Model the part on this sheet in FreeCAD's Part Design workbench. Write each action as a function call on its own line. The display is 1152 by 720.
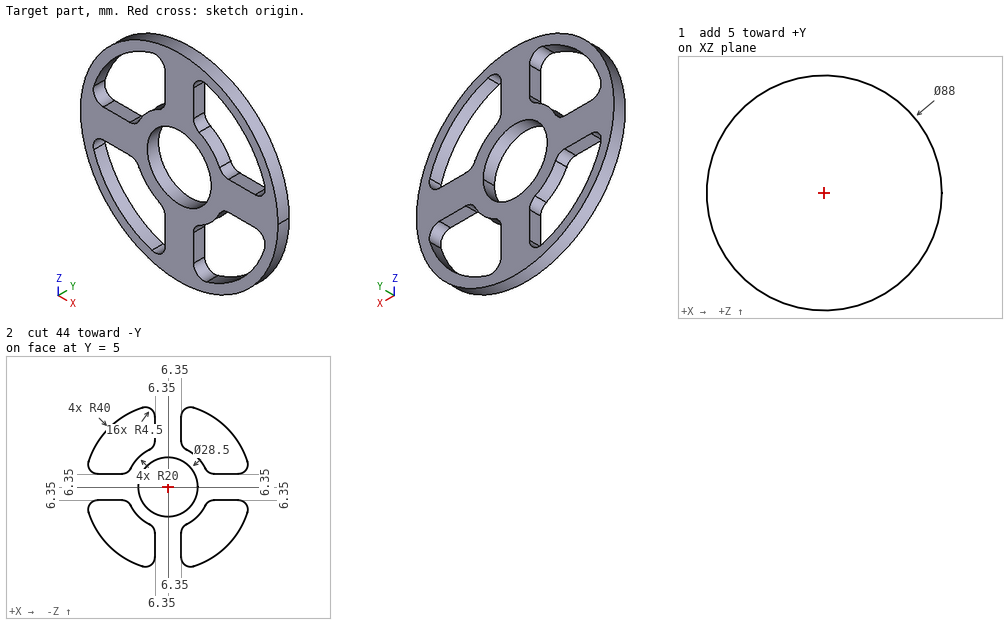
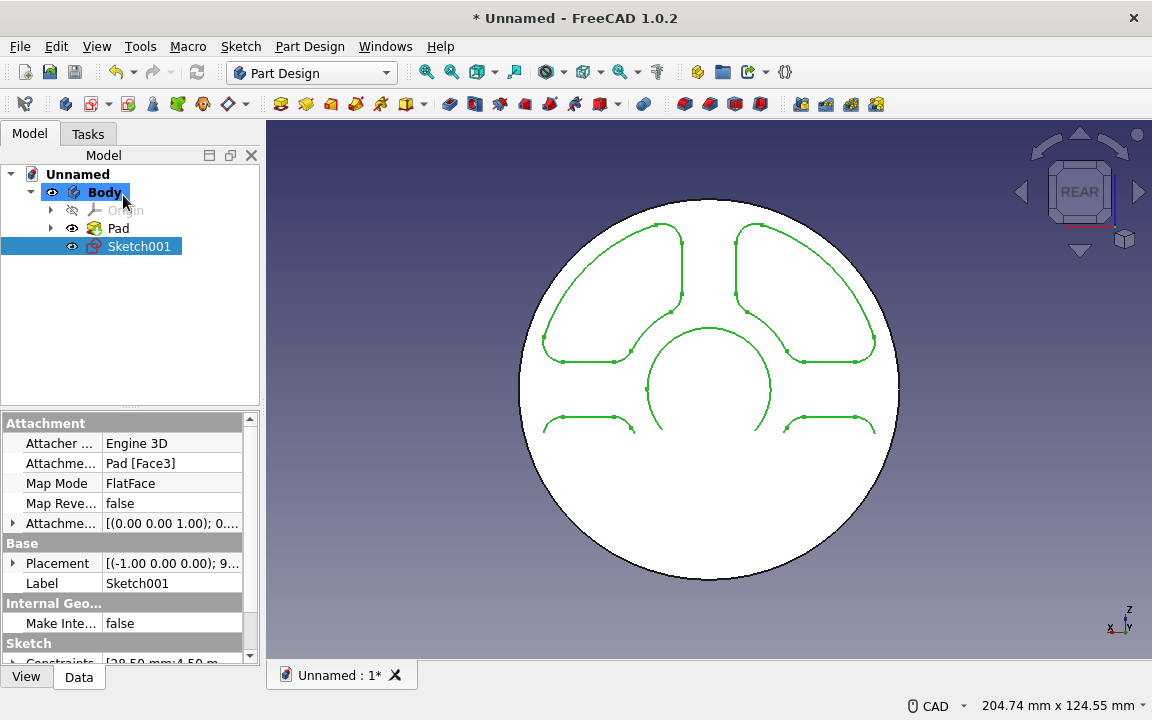
click(450, 104)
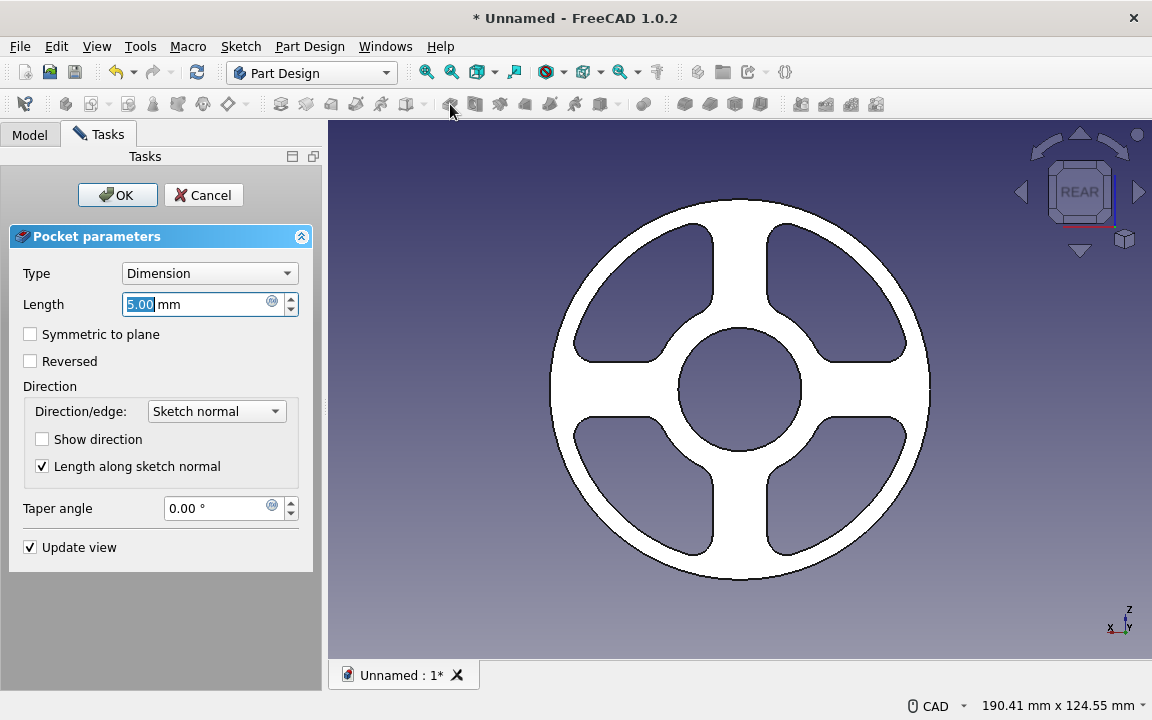
text(44)
key(Tab)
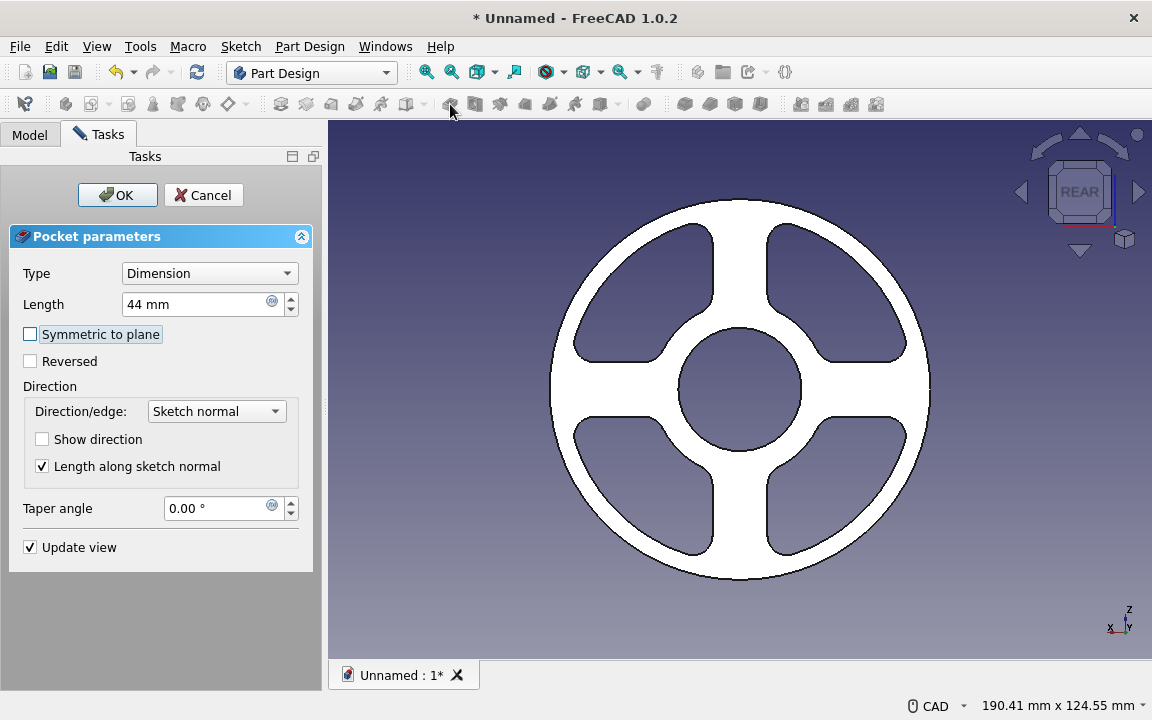
click(118, 195)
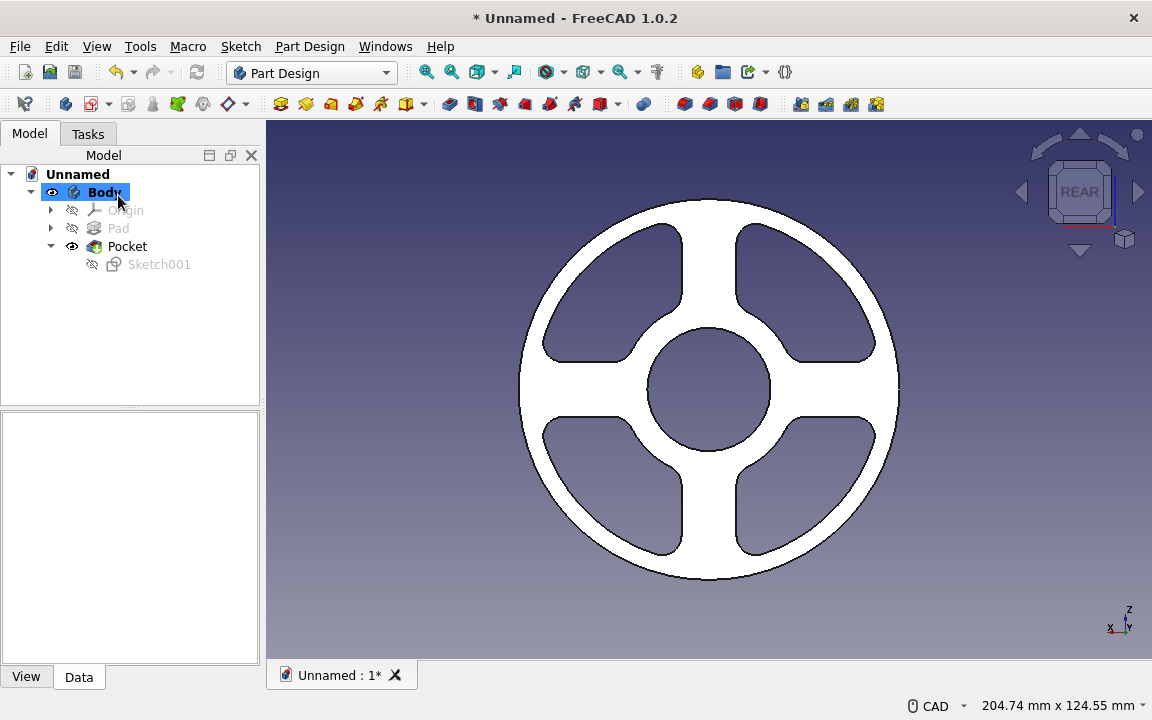
key(0)